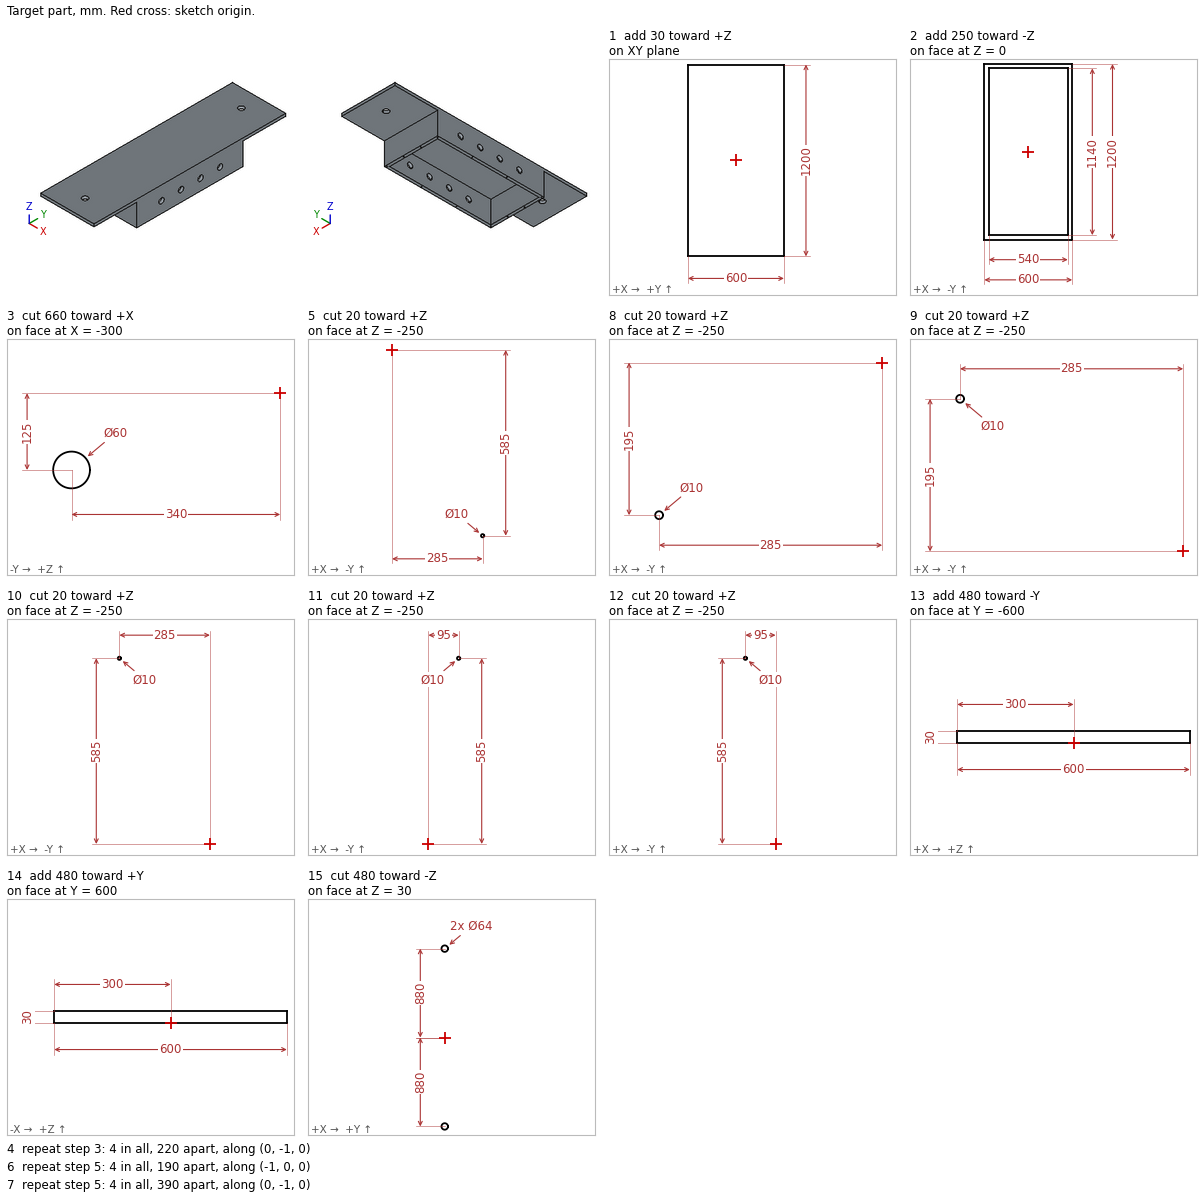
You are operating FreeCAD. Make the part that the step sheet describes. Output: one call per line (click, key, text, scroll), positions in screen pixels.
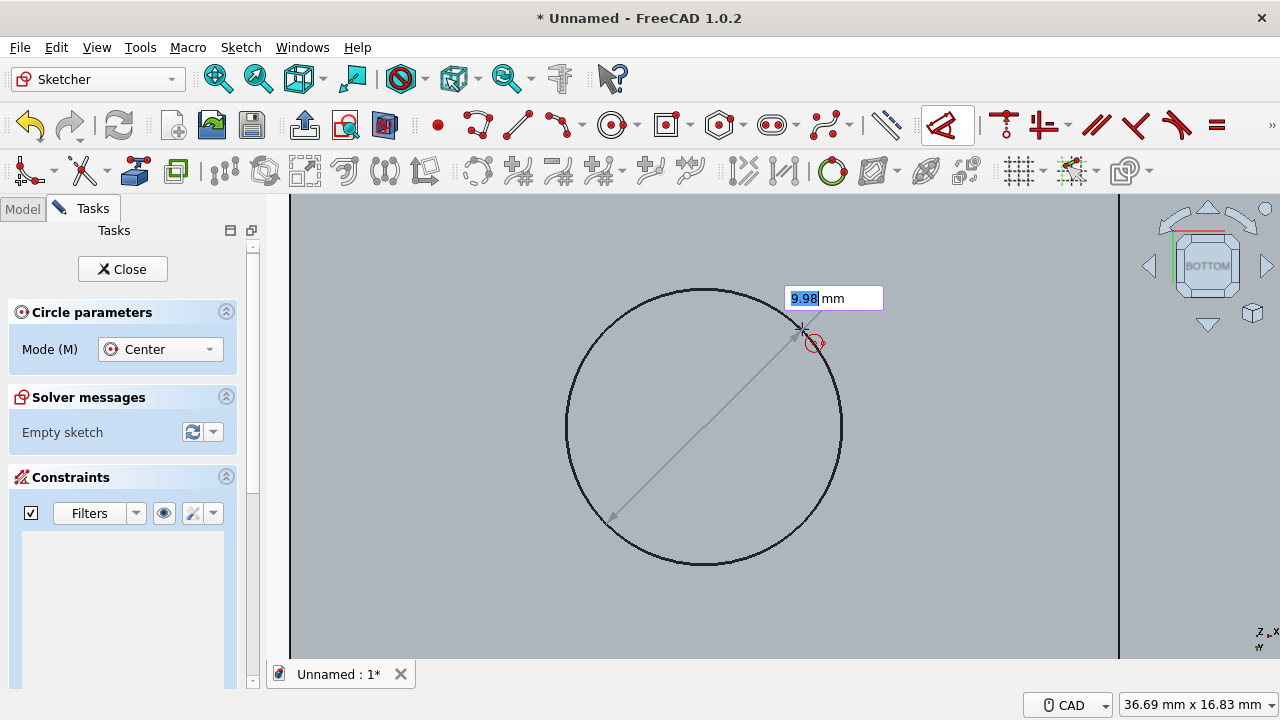
text(10)
key(Return)
key(Escape)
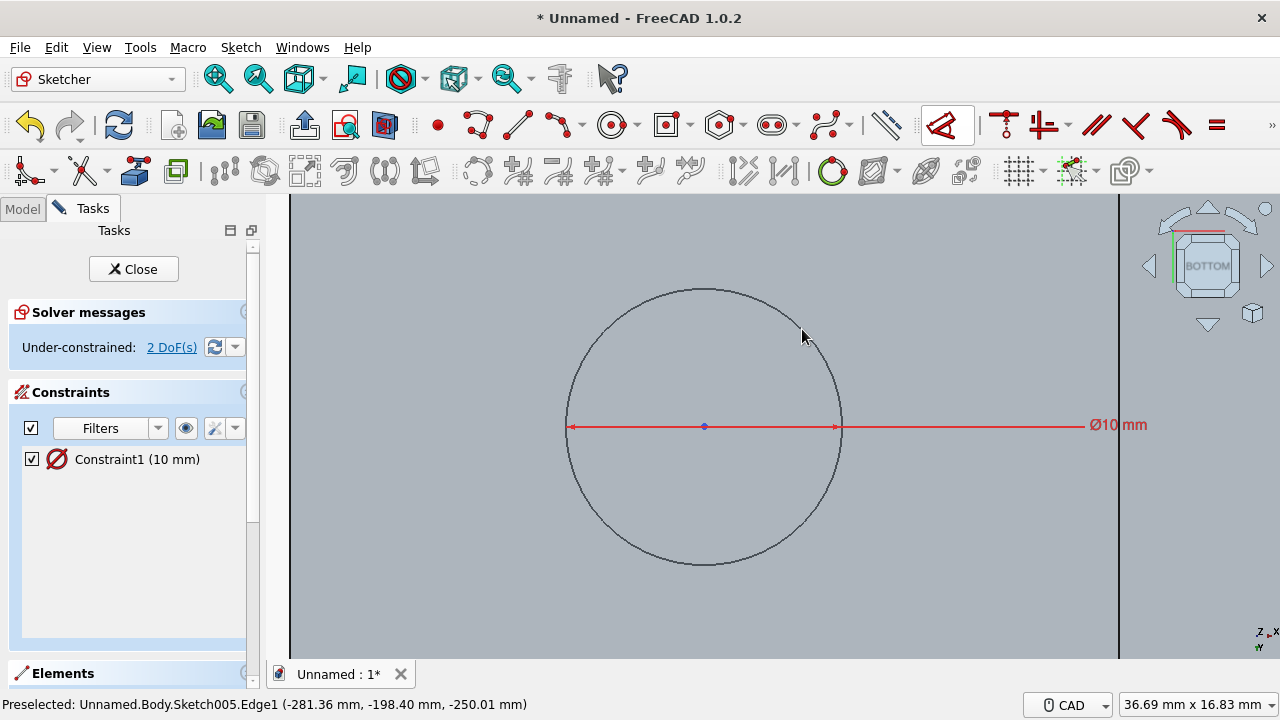
click(704, 427)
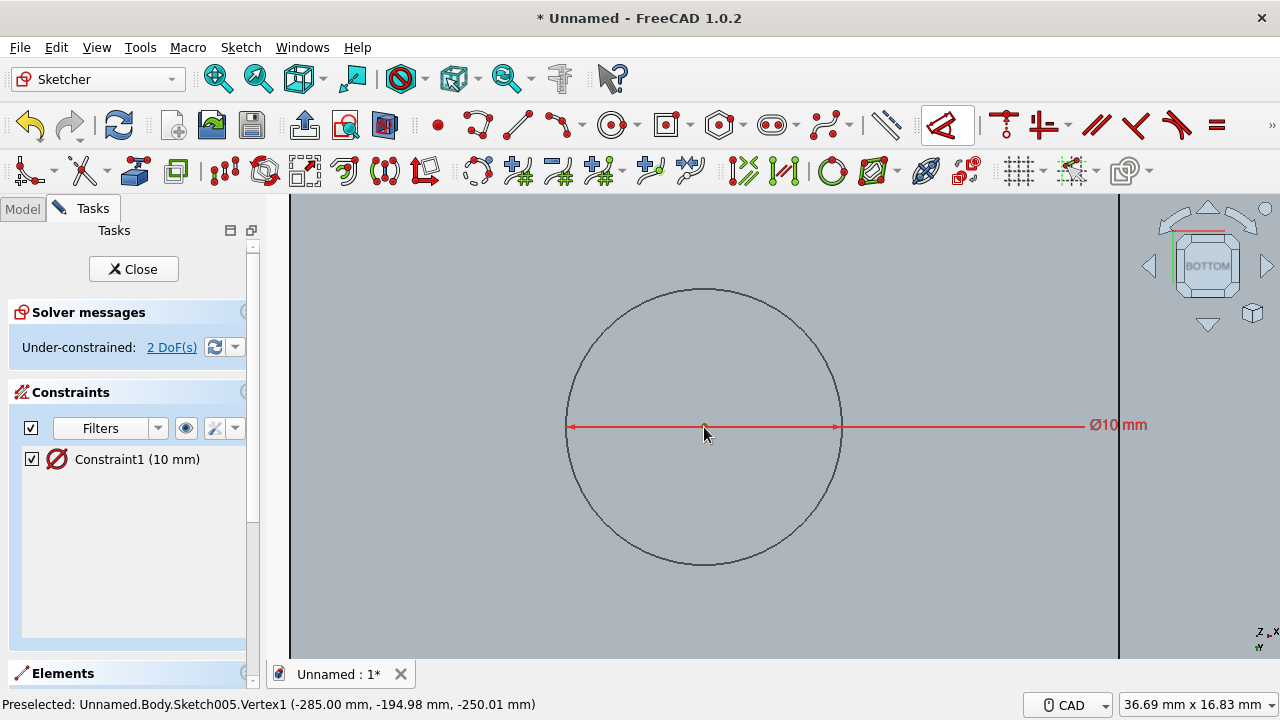
key(l)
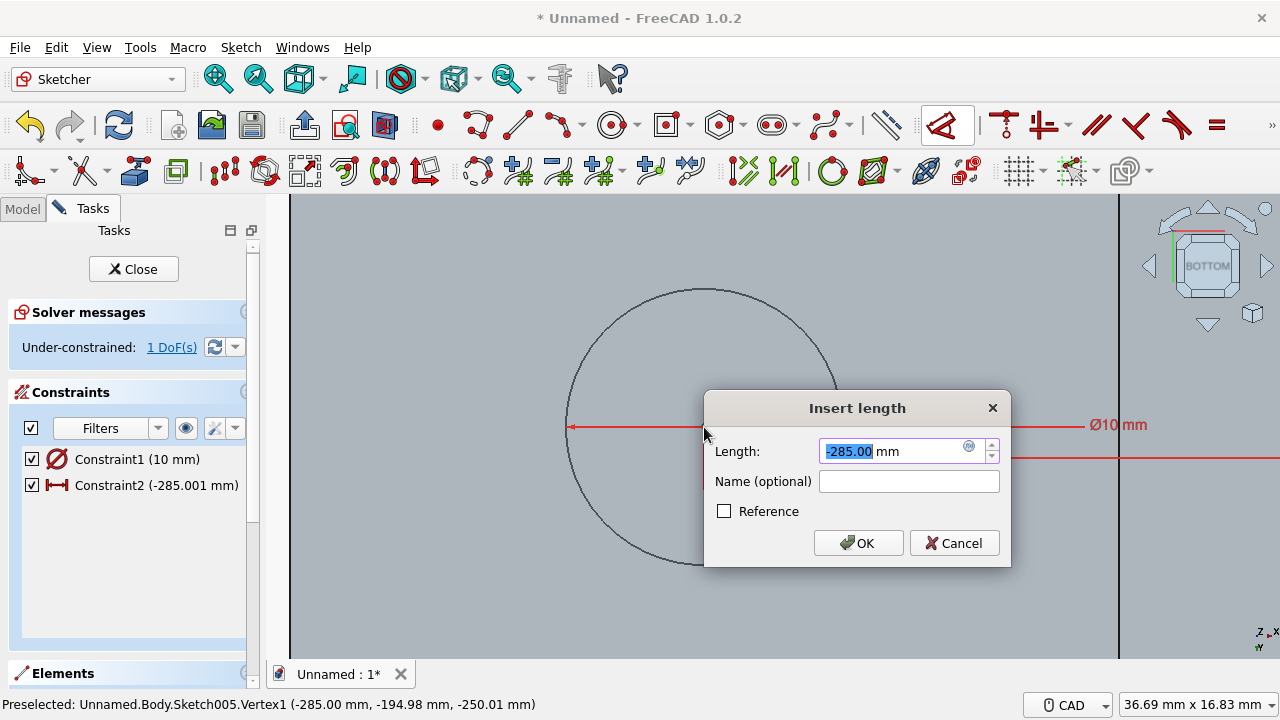
text(-285)
key(Return)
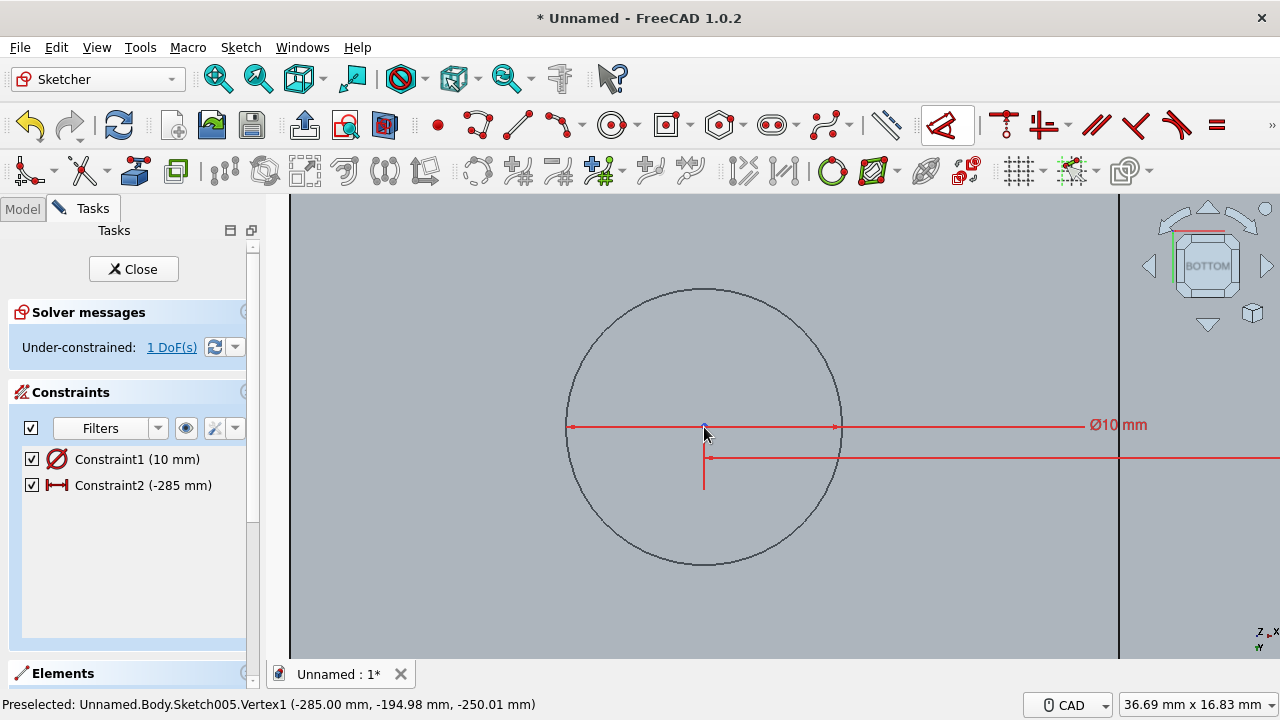
click(704, 427)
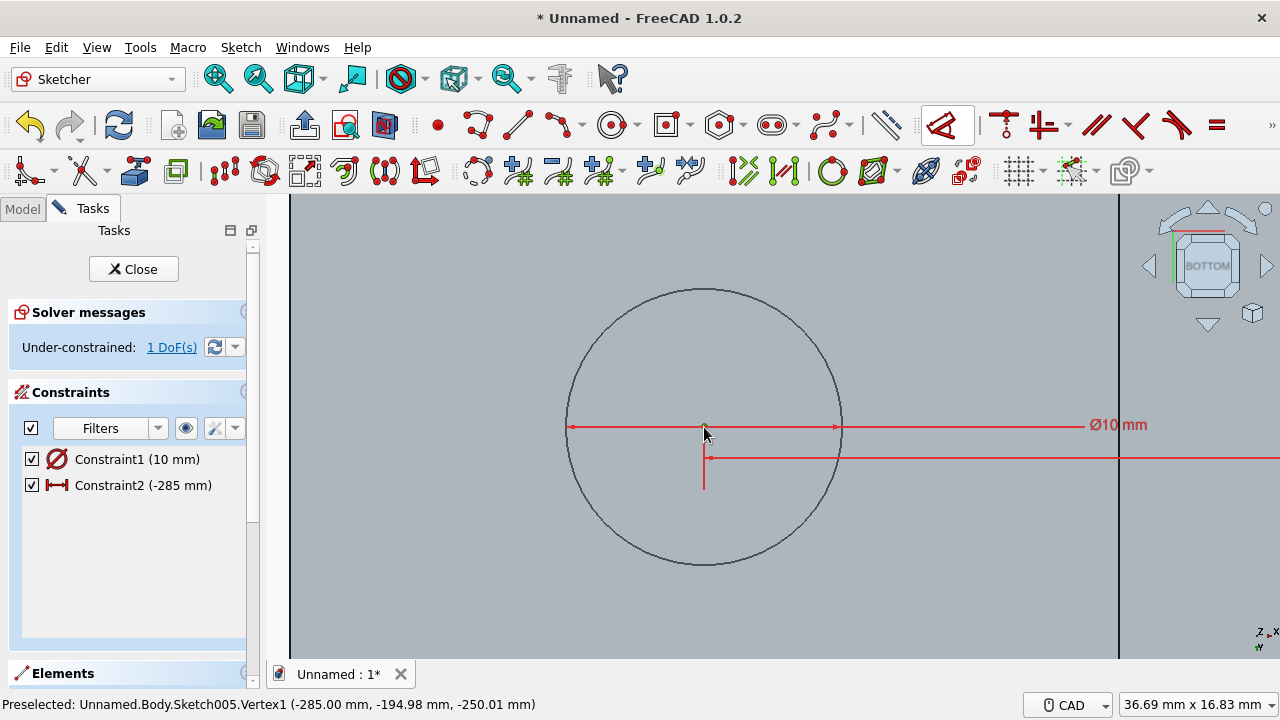
key(i)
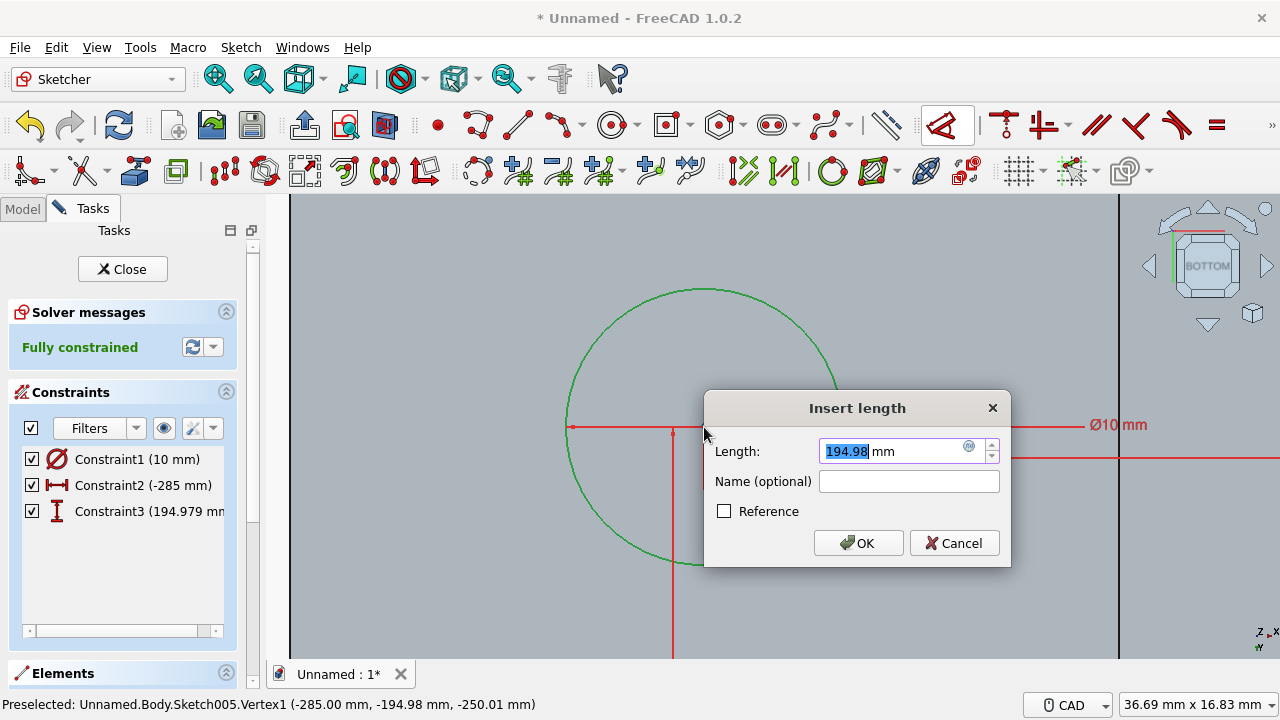
text(195)
key(Return)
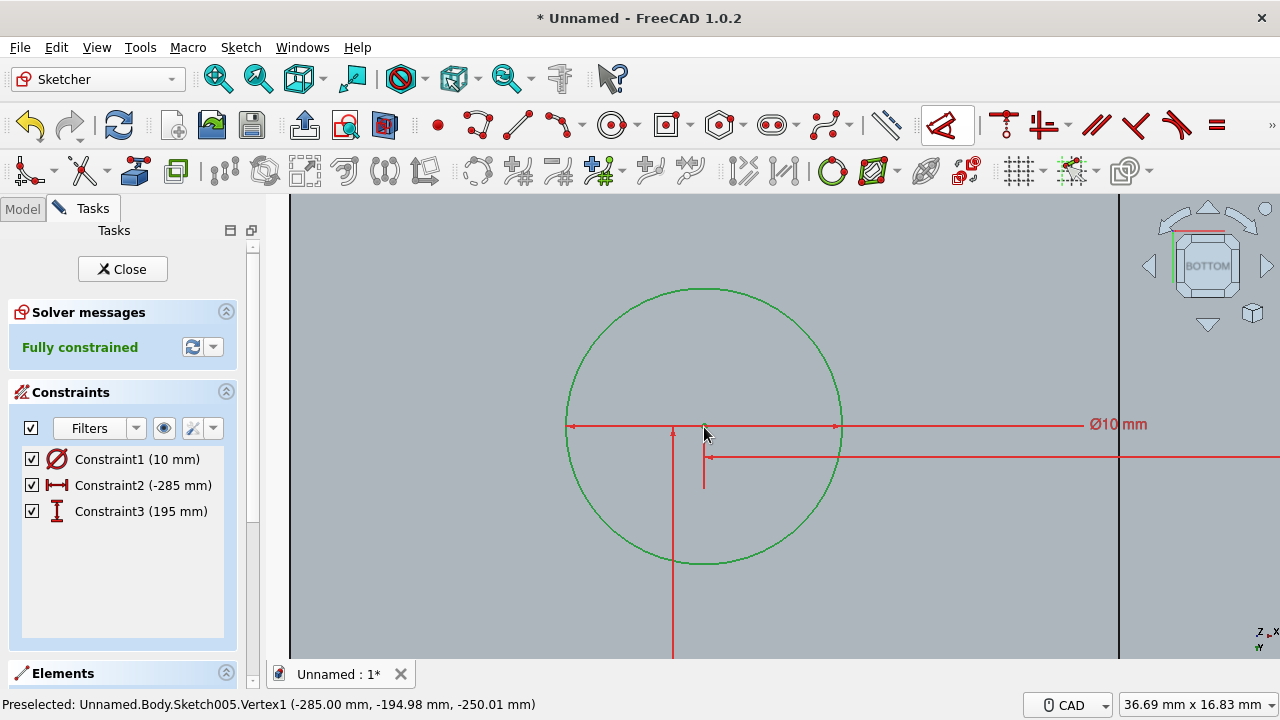
click(123, 269)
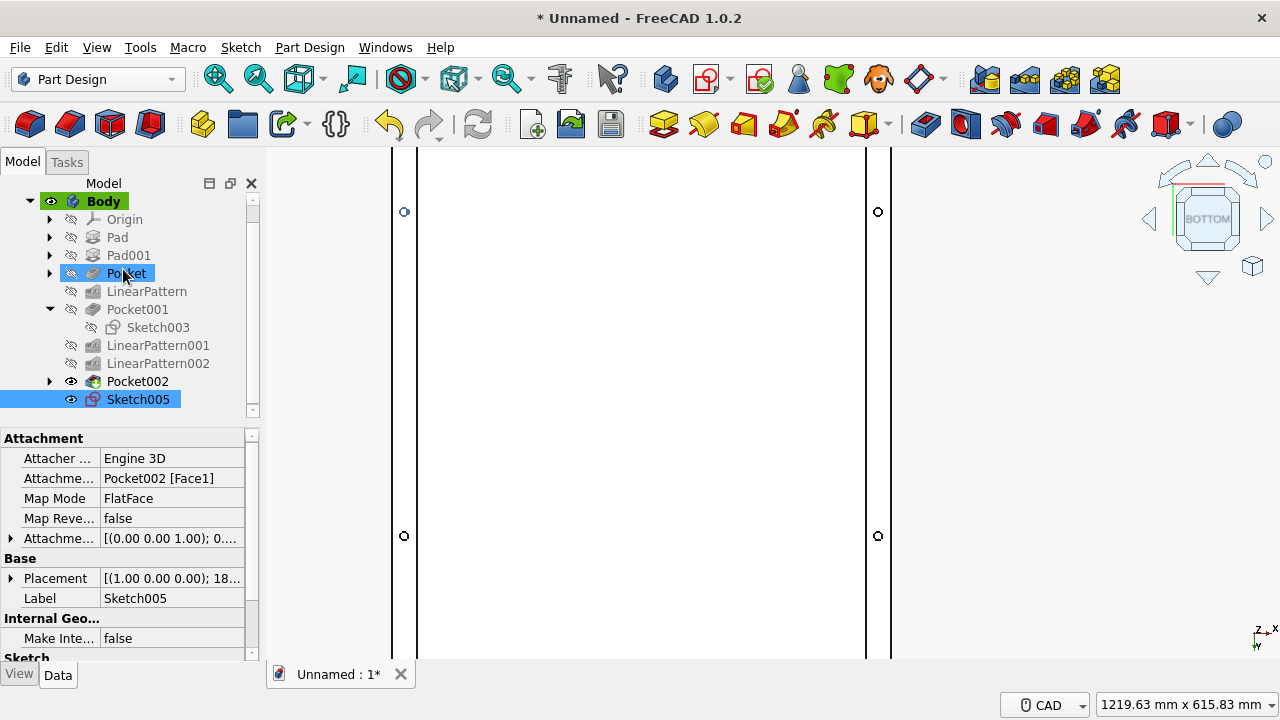
click(926, 124)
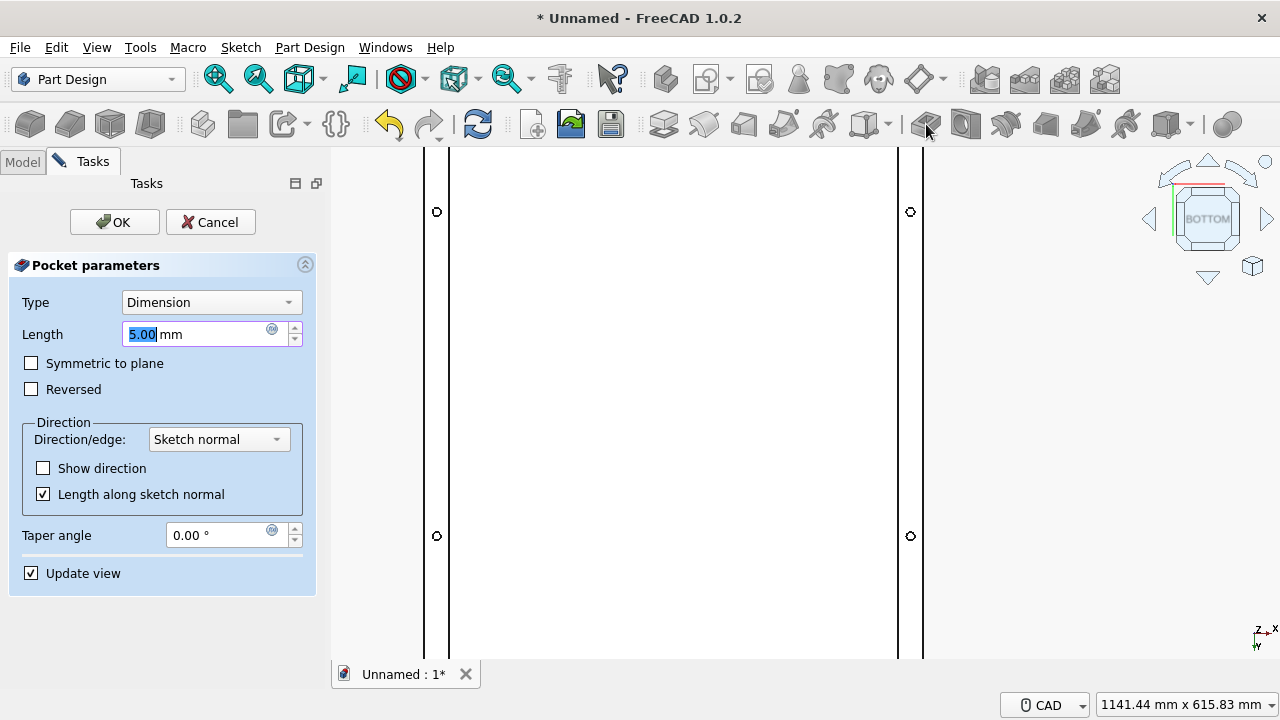
text(20)
key(Tab)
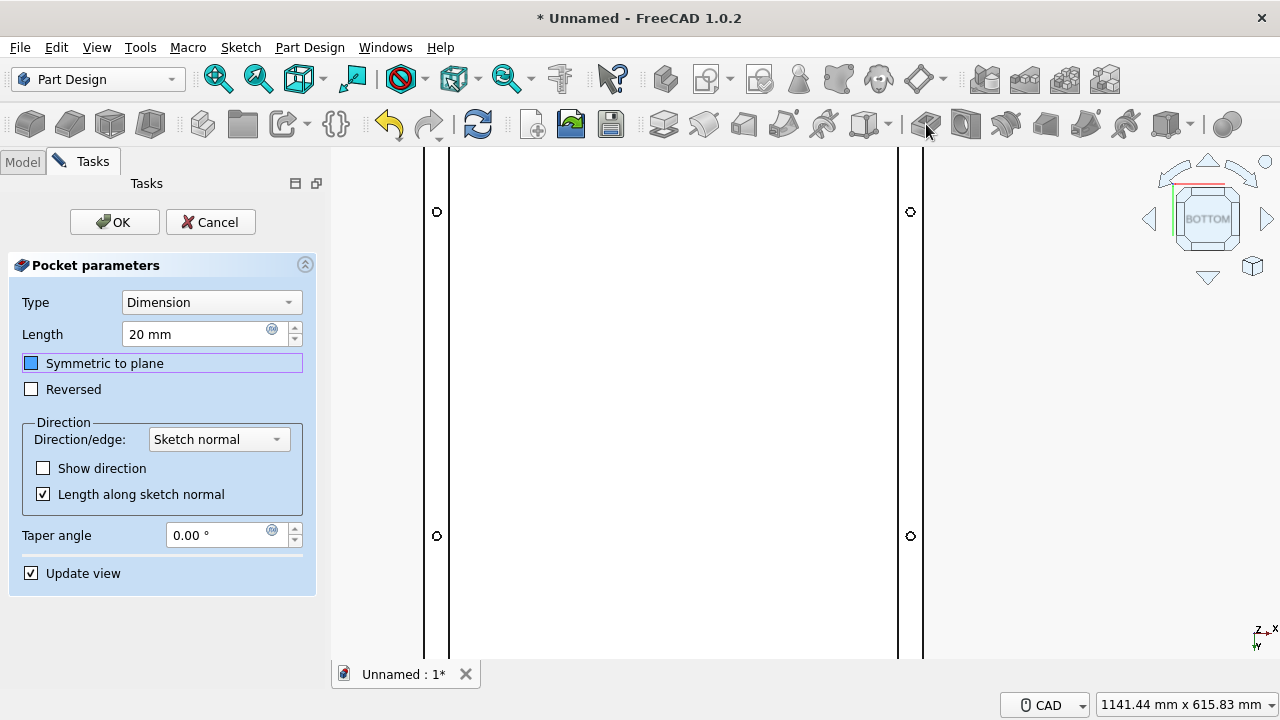
click(115, 222)